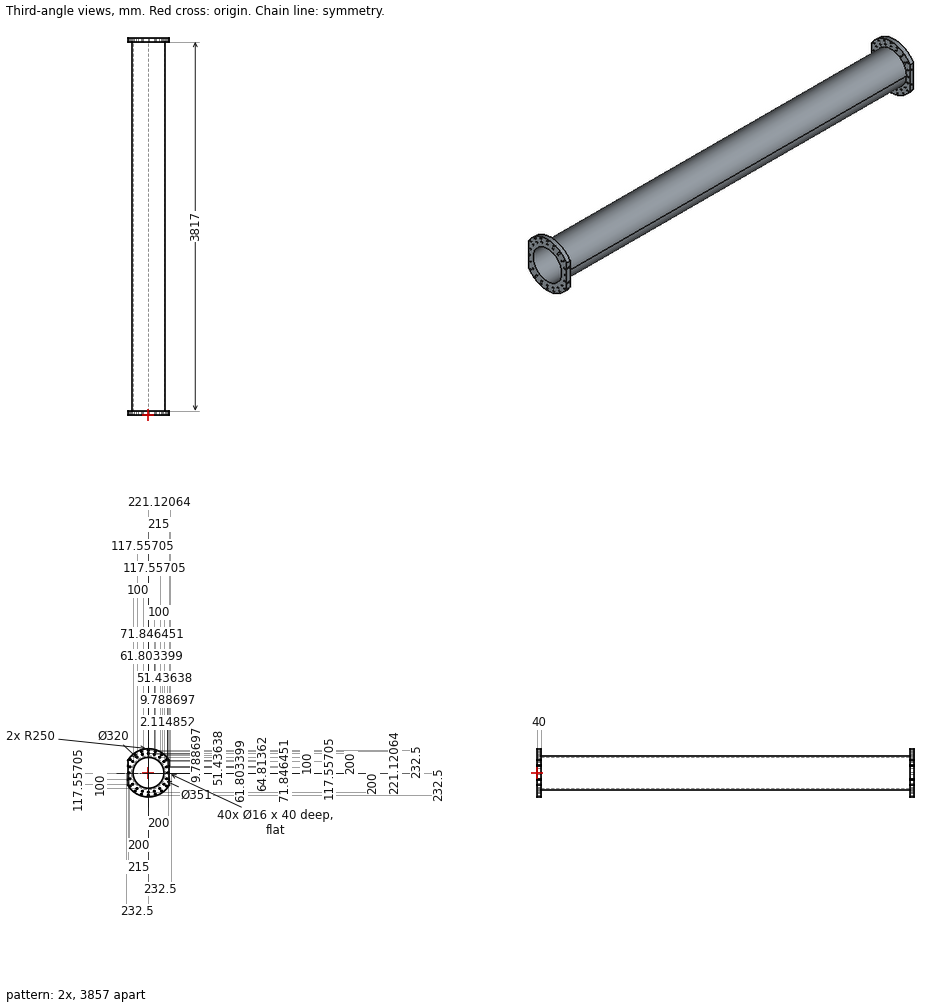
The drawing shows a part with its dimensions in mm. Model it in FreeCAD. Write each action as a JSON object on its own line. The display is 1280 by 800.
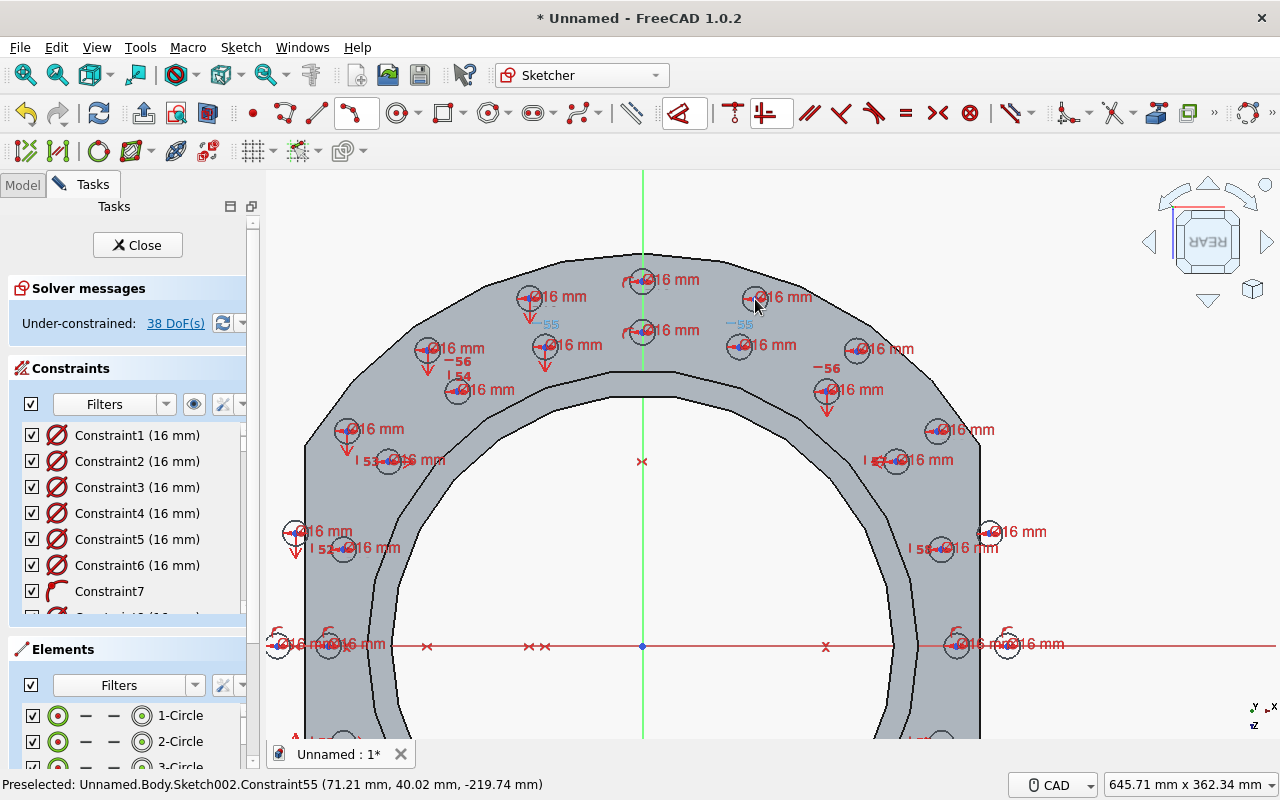
{"action": "left_click", "coordinate": [755, 299]}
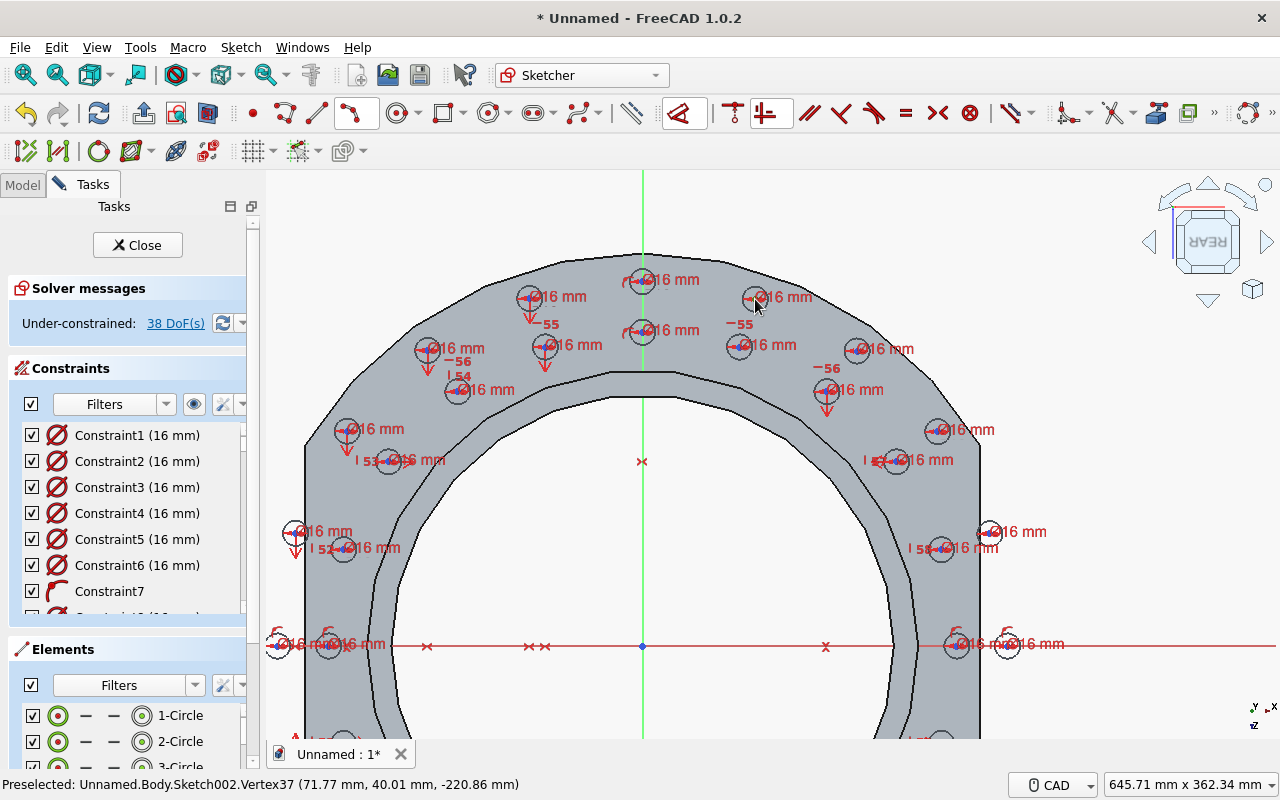
{"action": "left_click", "coordinate": [411, 646]}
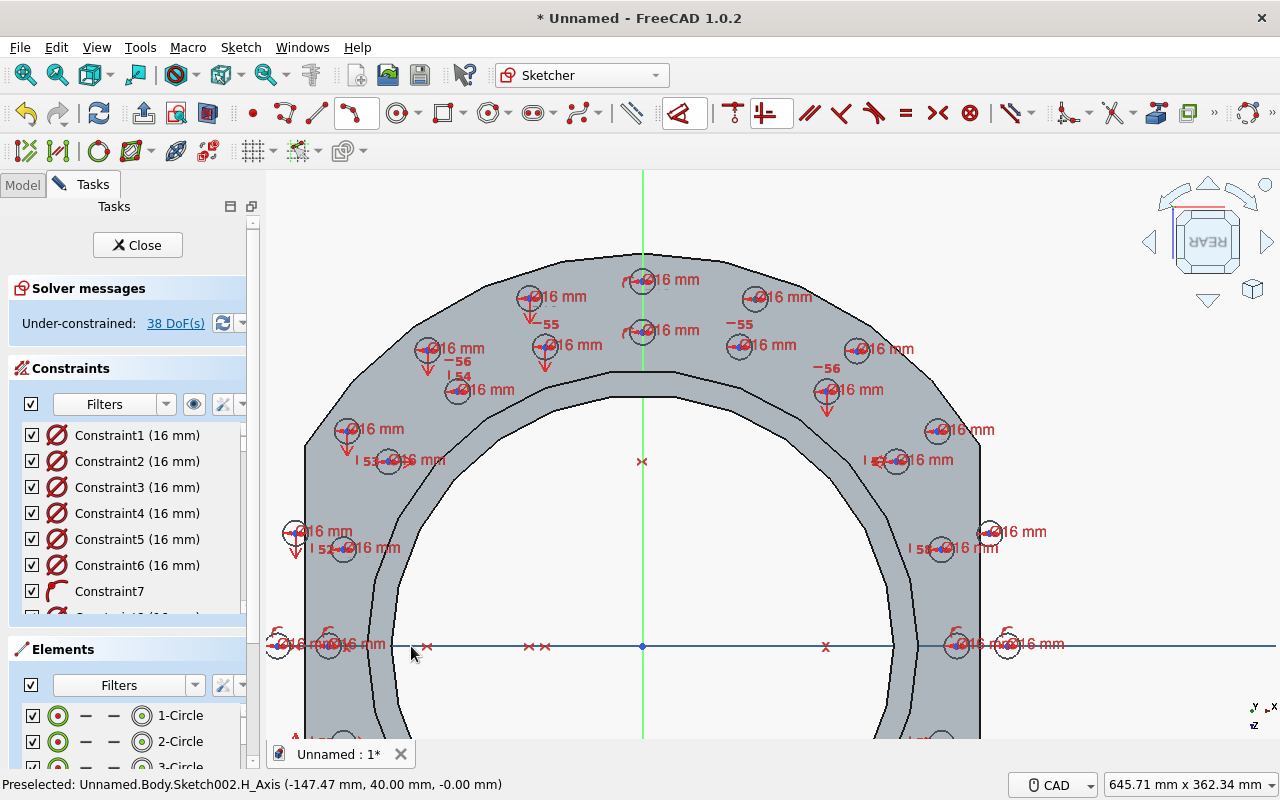
{"action": "left_click", "coordinate": [938, 114]}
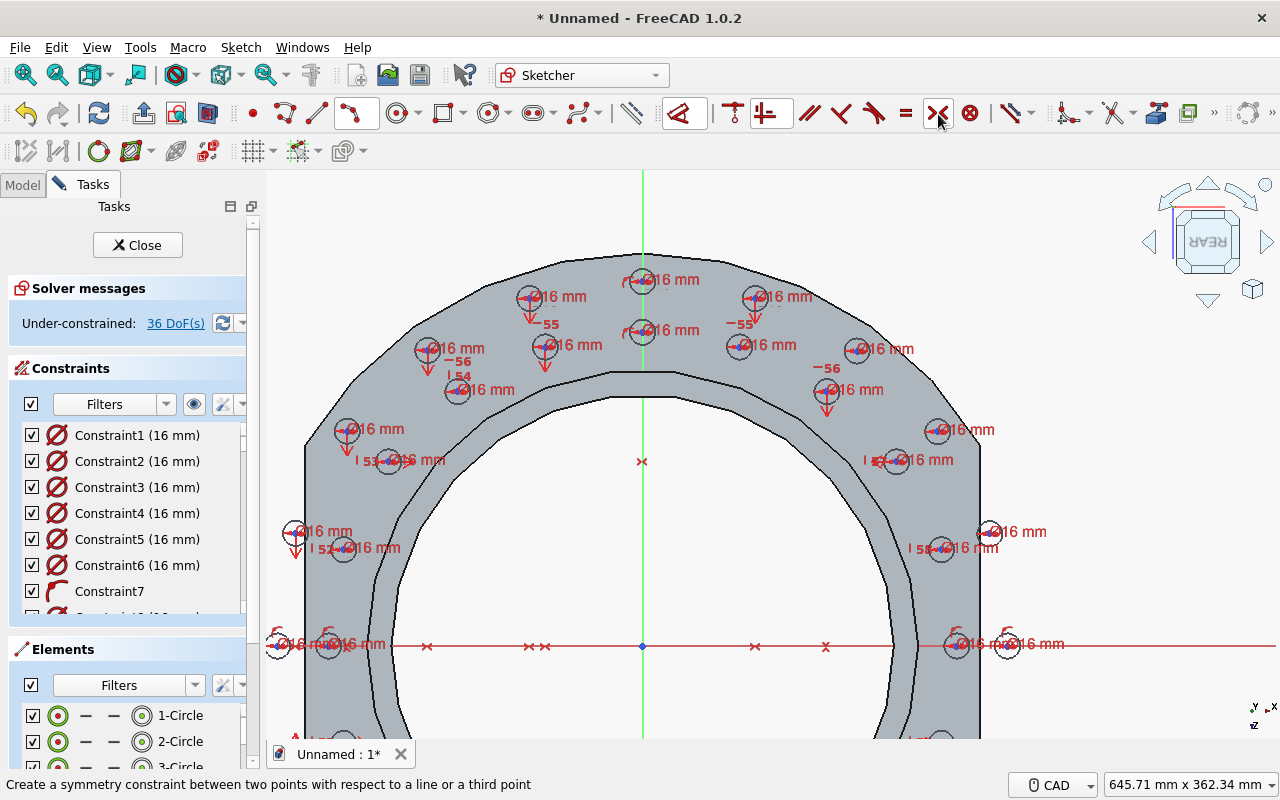
{"action": "scroll", "coordinate": [755, 298], "scroll_direction": "down", "scroll_amount": 4}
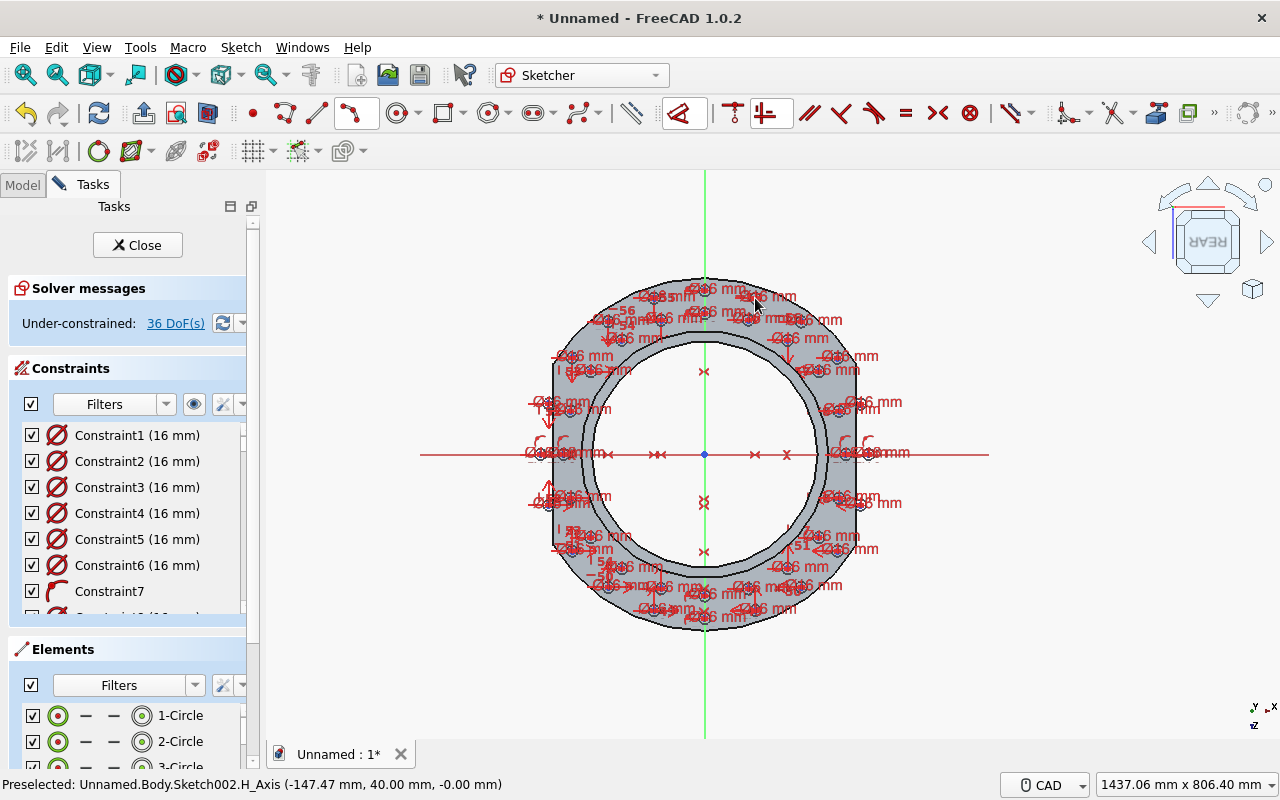
{"action": "left_click", "coordinate": [801, 587]}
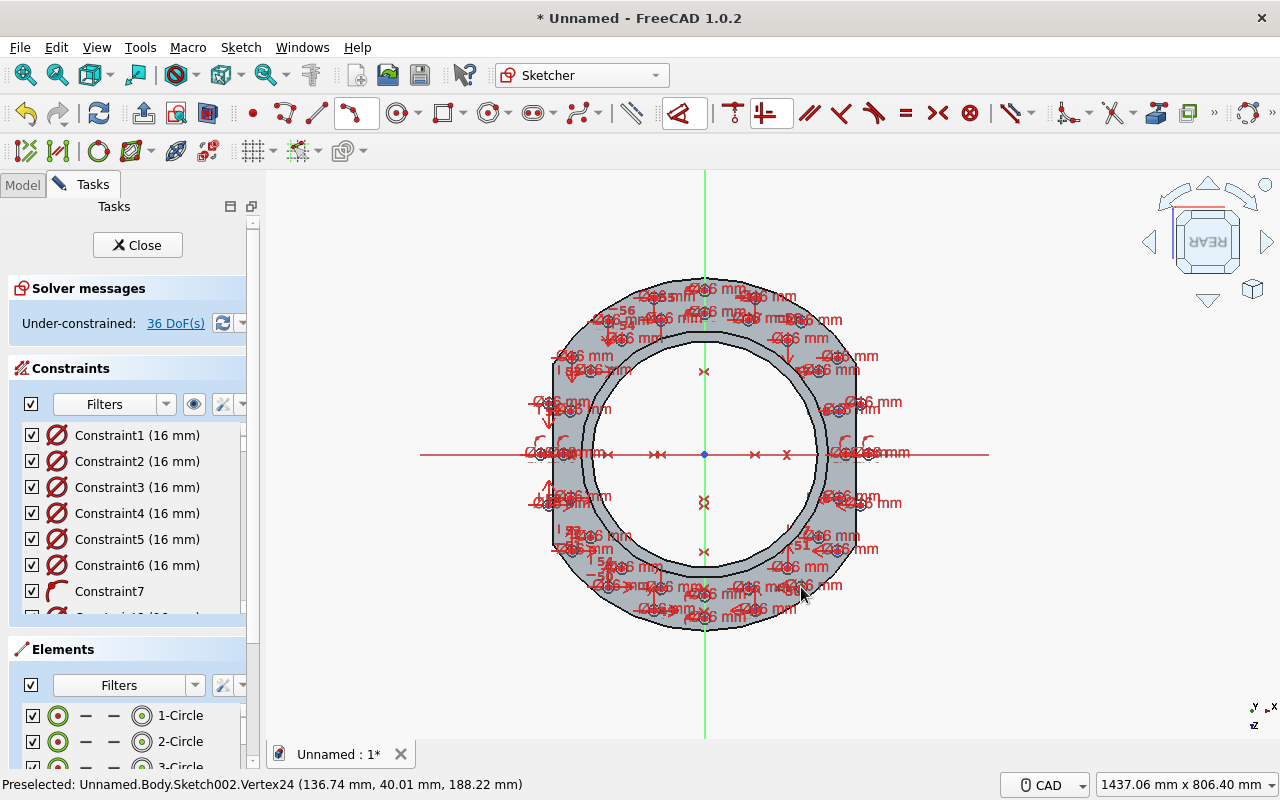
{"action": "left_click", "coordinate": [799, 324]}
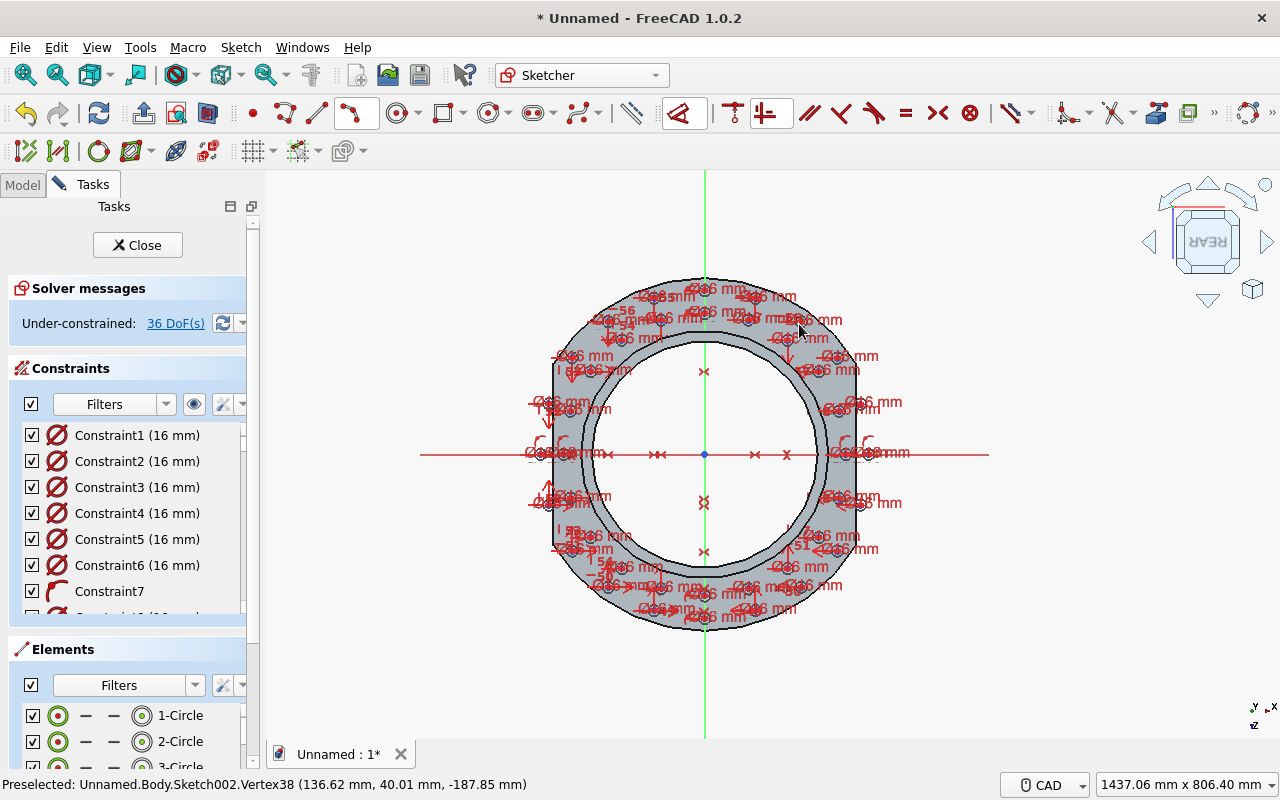
{"action": "left_click", "coordinate": [470, 454]}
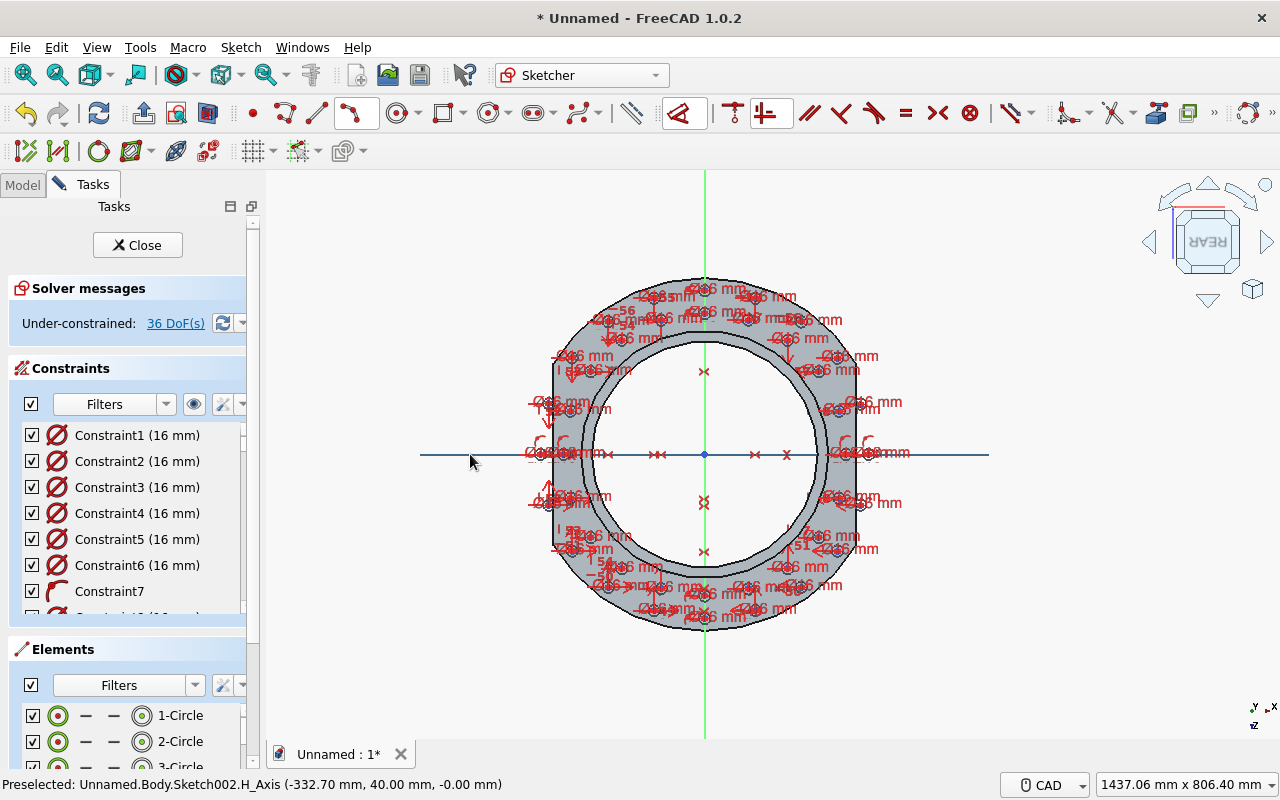
{"action": "left_click", "coordinate": [938, 114]}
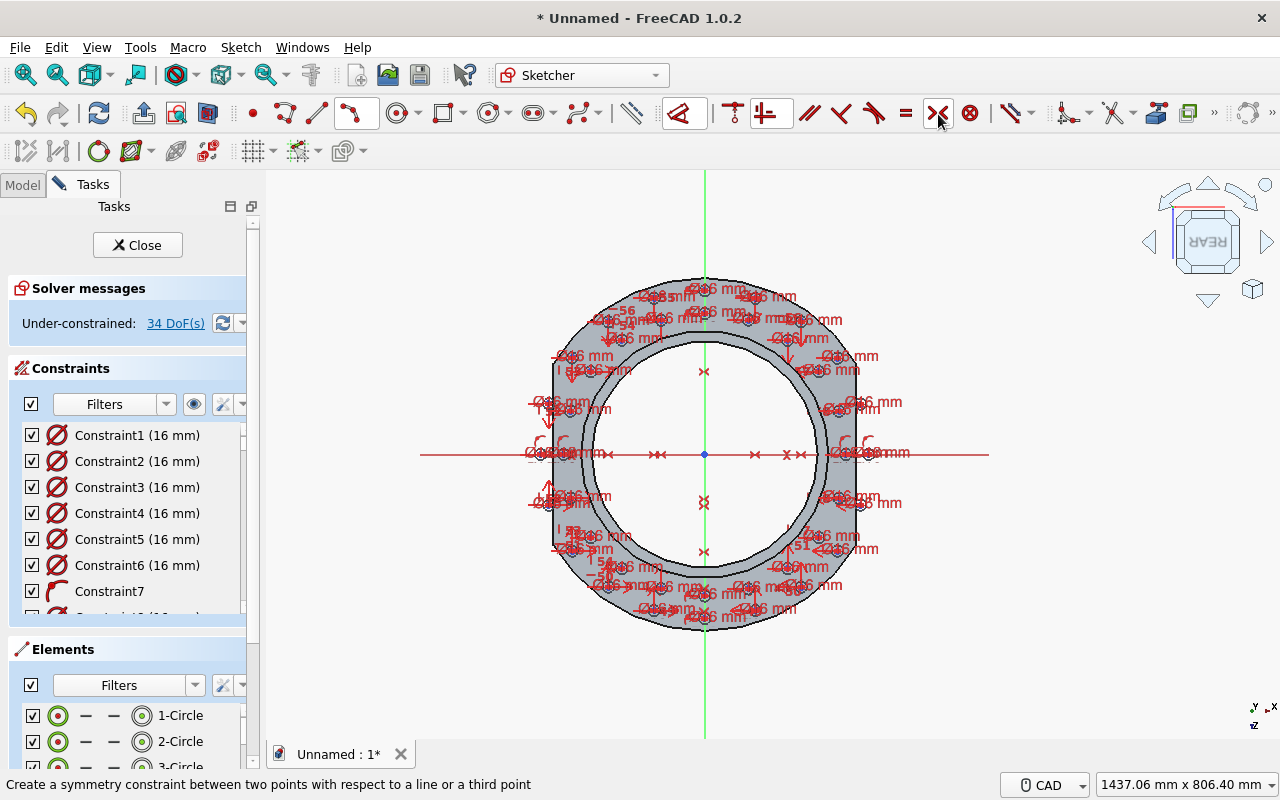
{"action": "left_click", "coordinate": [837, 551]}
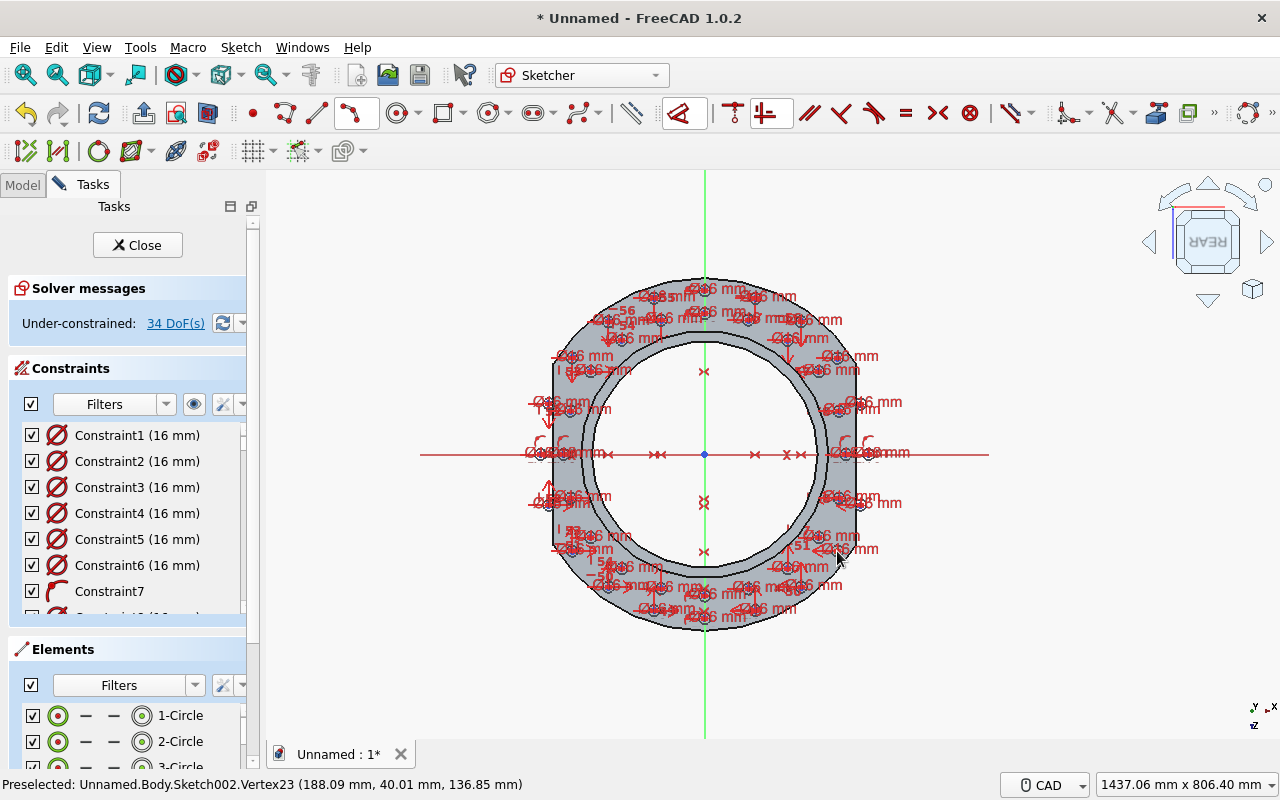
{"action": "left_click", "coordinate": [837, 358]}